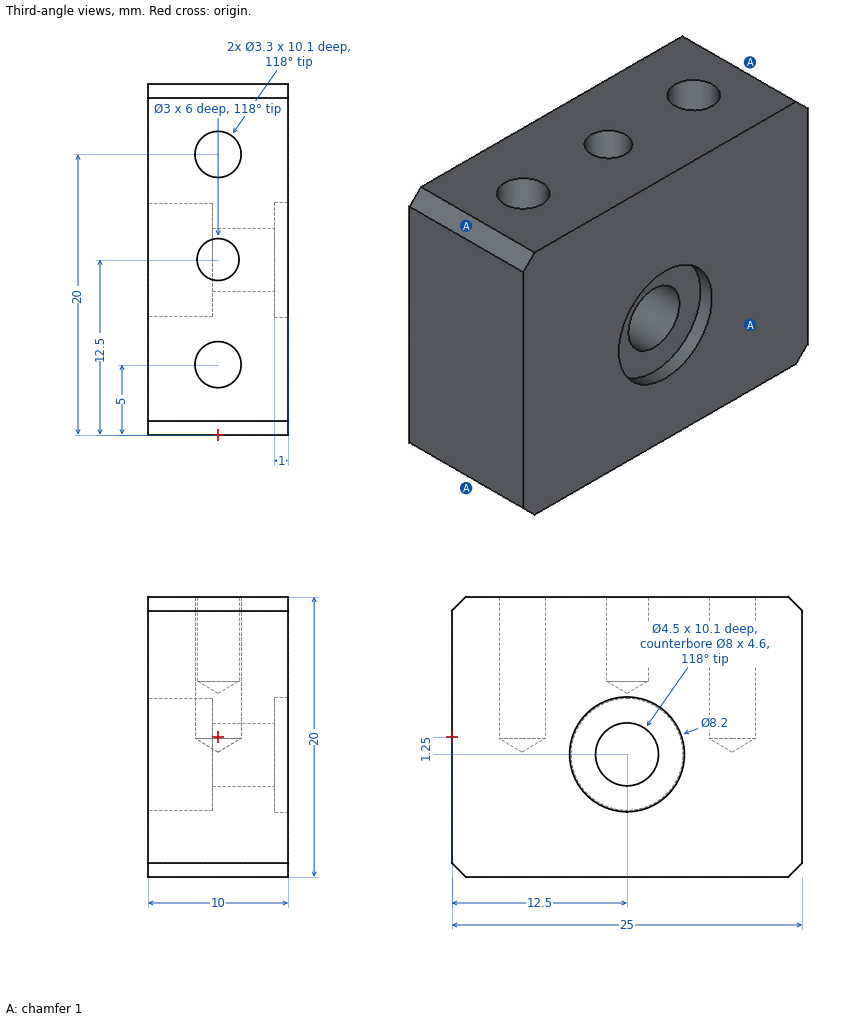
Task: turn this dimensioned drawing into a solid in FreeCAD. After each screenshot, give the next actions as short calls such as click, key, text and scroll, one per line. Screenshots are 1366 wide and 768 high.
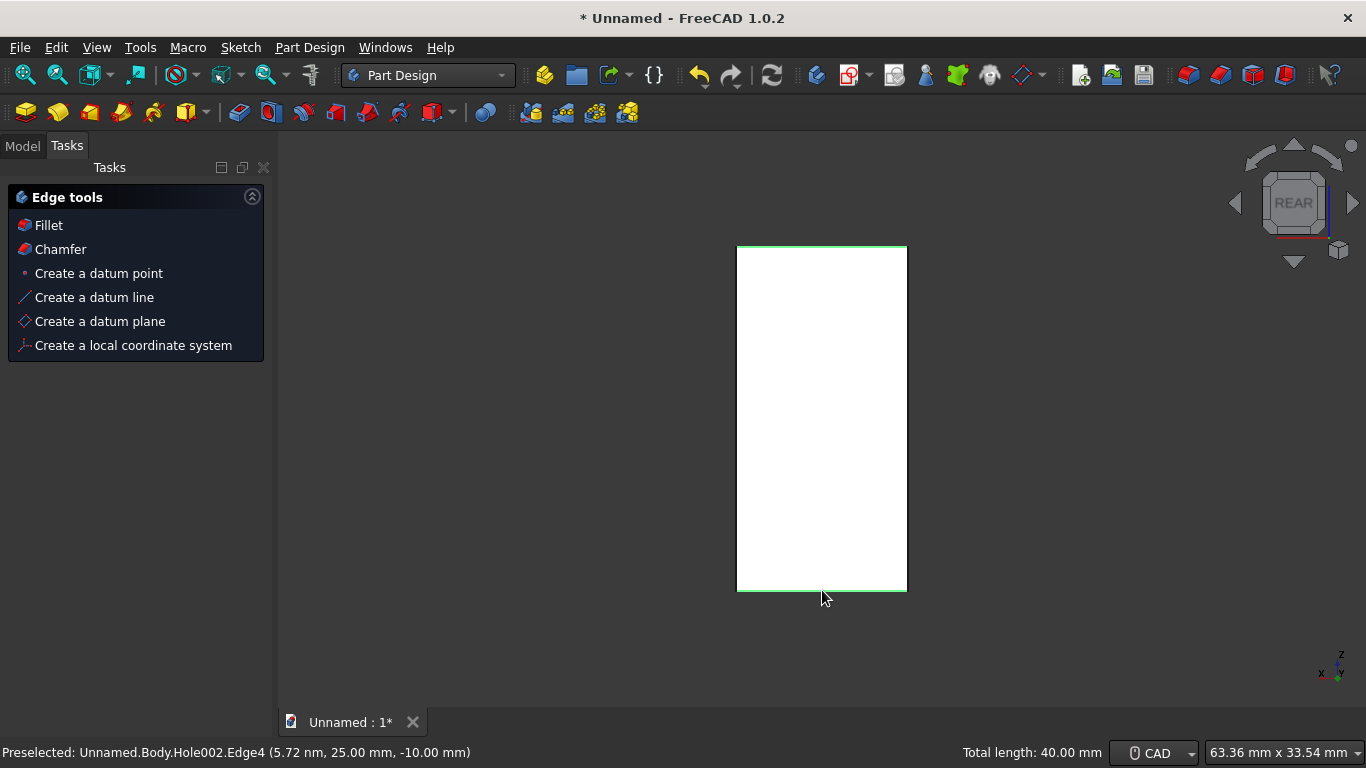
click(1222, 76)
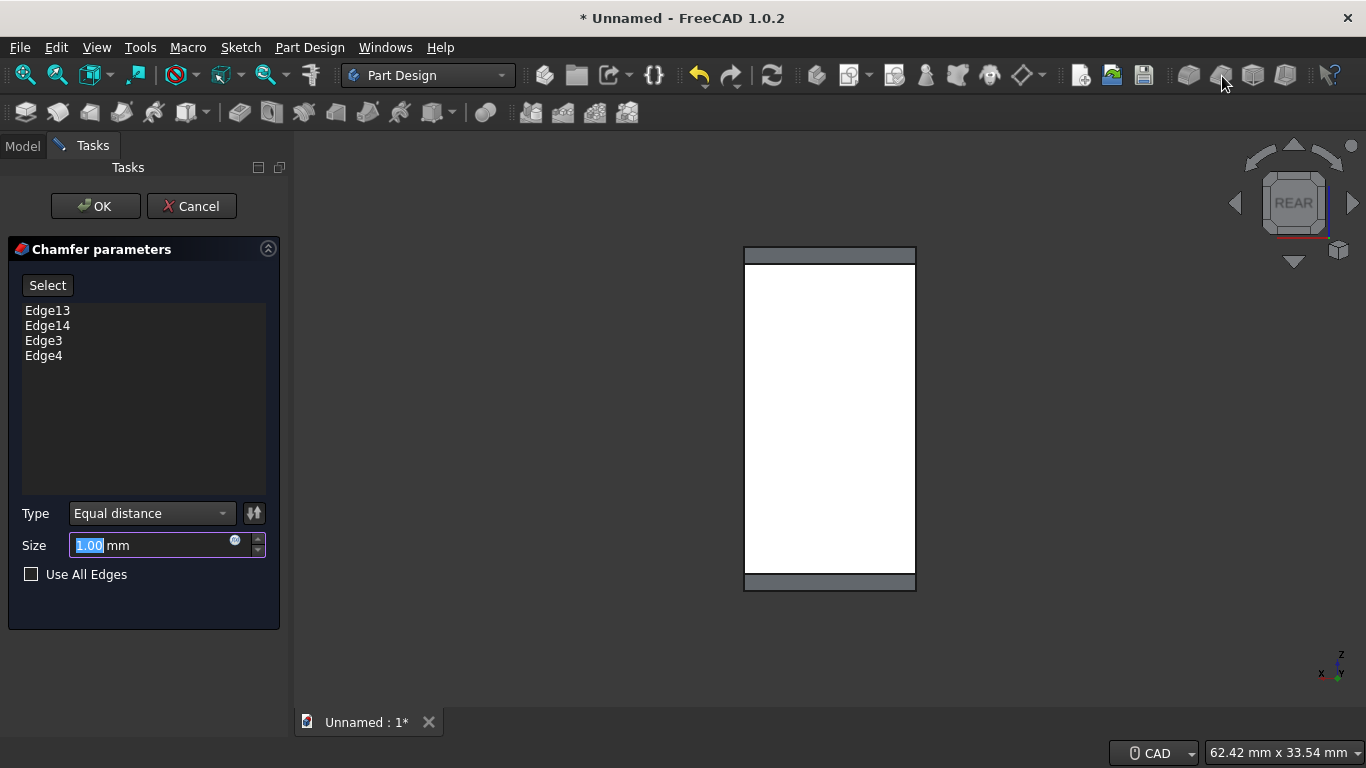
text(1)
key(Tab)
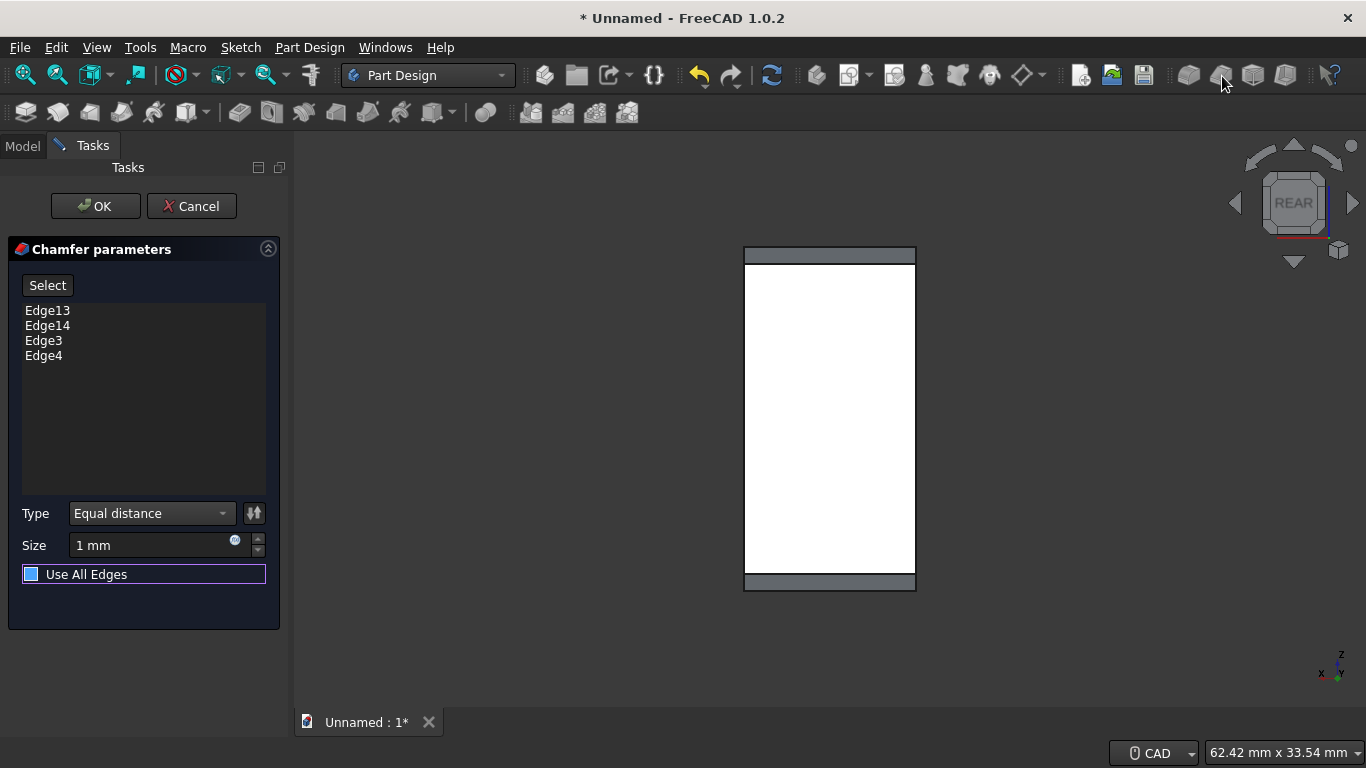
click(96, 206)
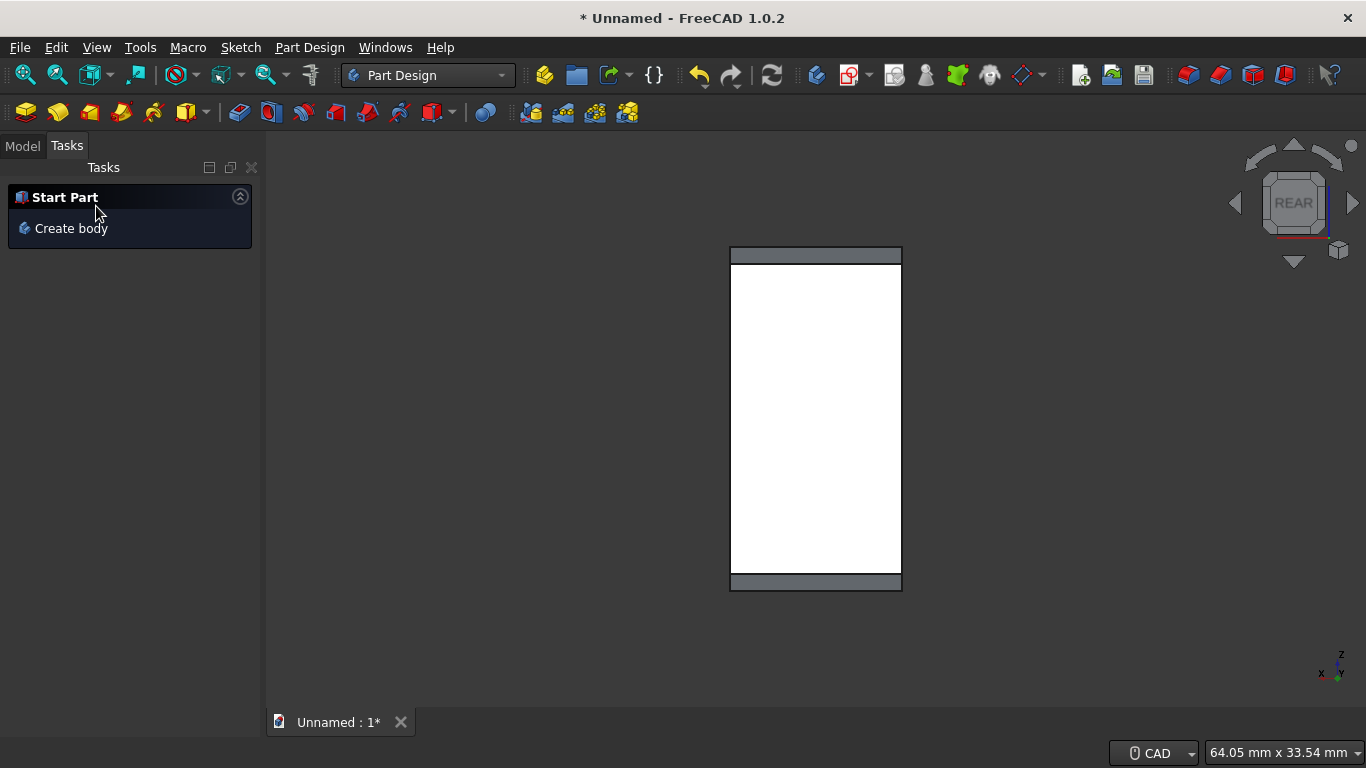
key(0)